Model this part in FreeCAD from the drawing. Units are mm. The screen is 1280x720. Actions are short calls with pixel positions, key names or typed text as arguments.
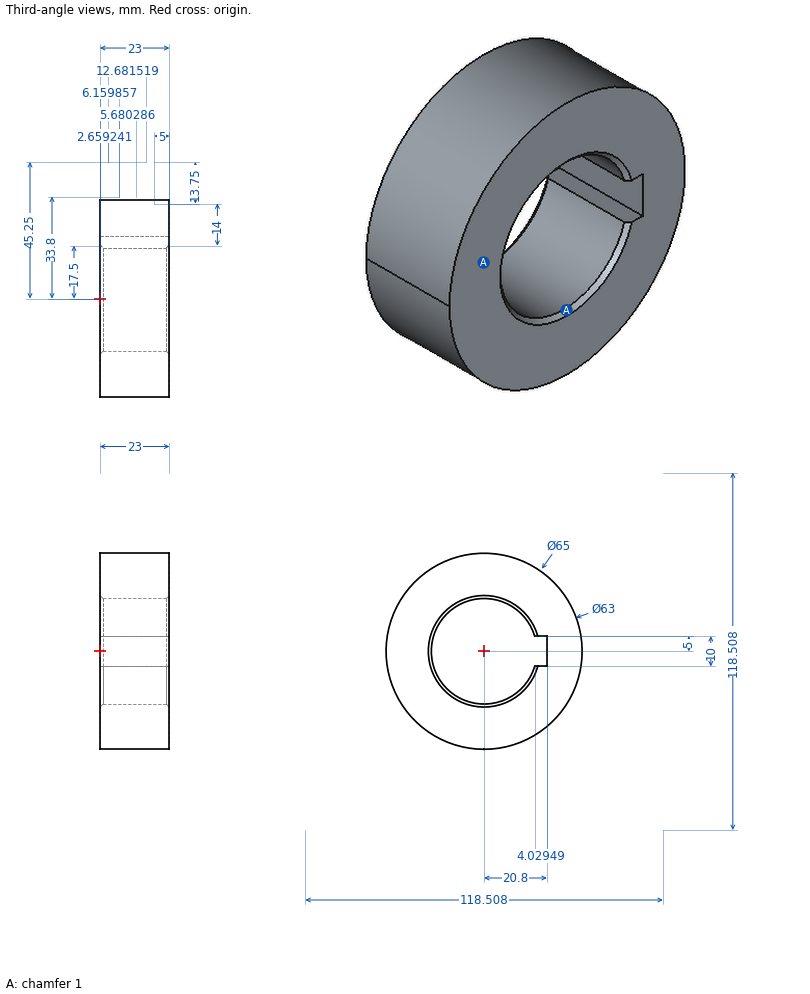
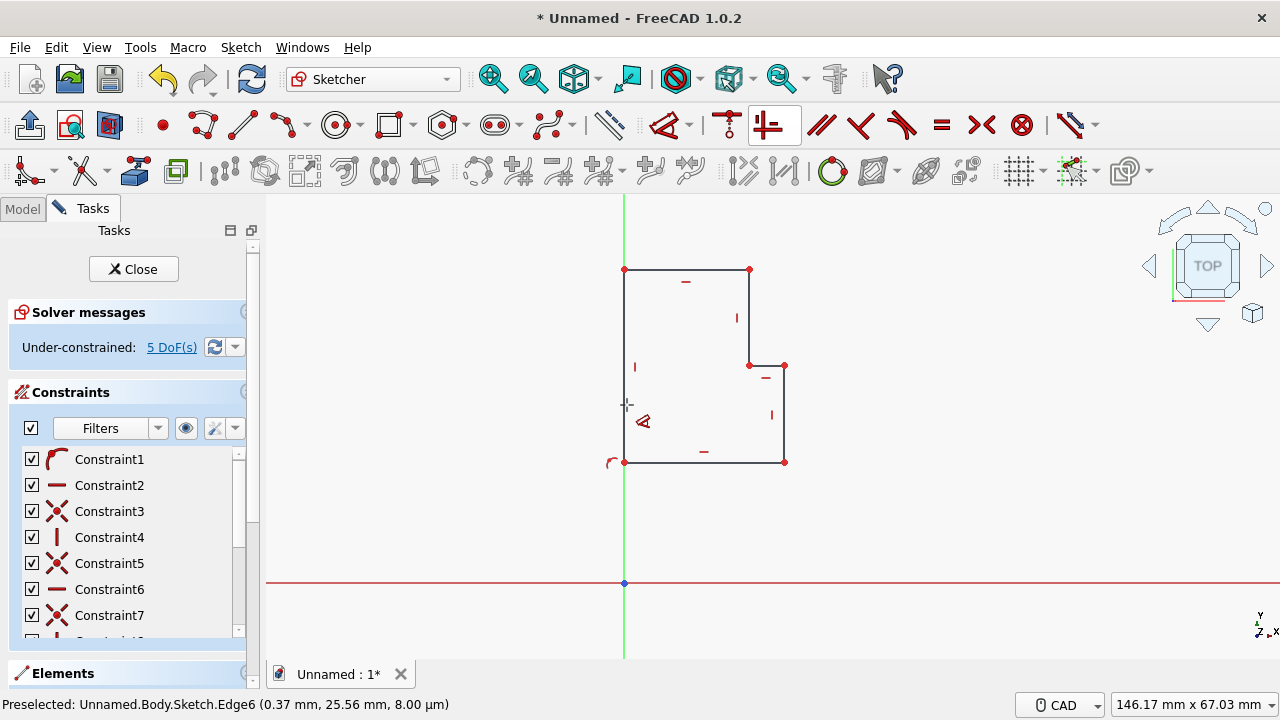
scroll(773, 366, up, 2)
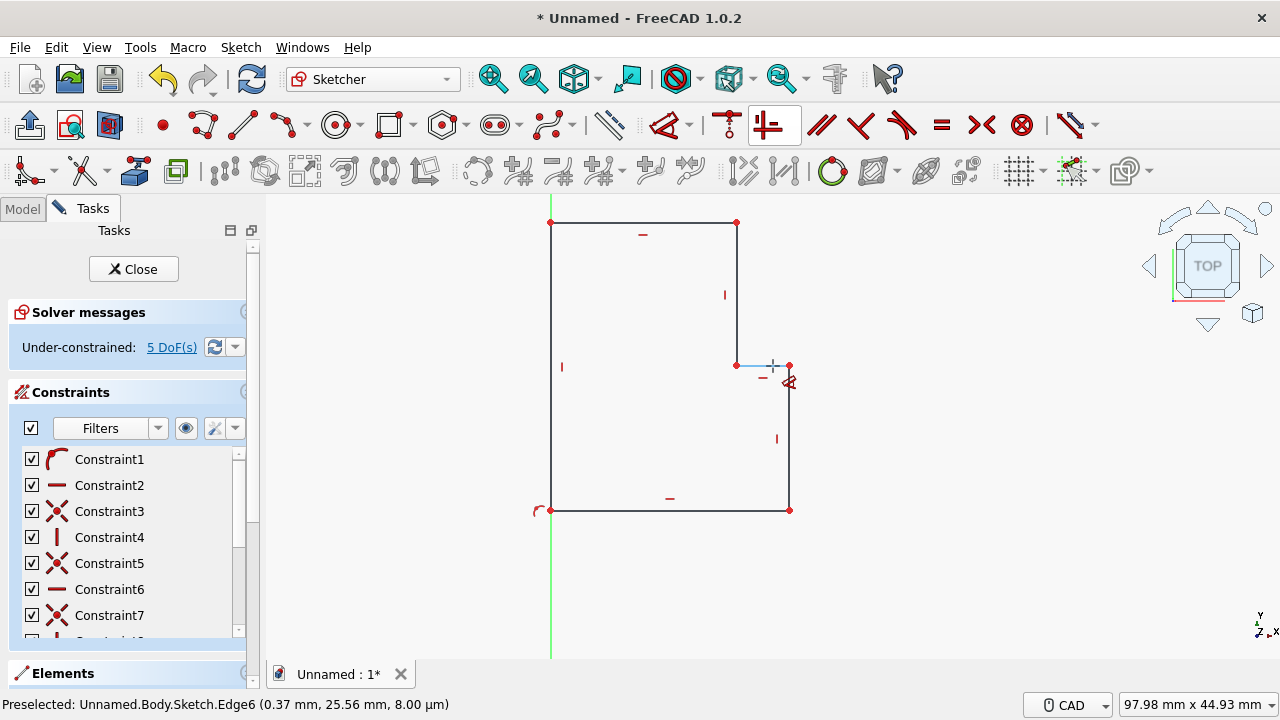
click(773, 366)
click(763, 332)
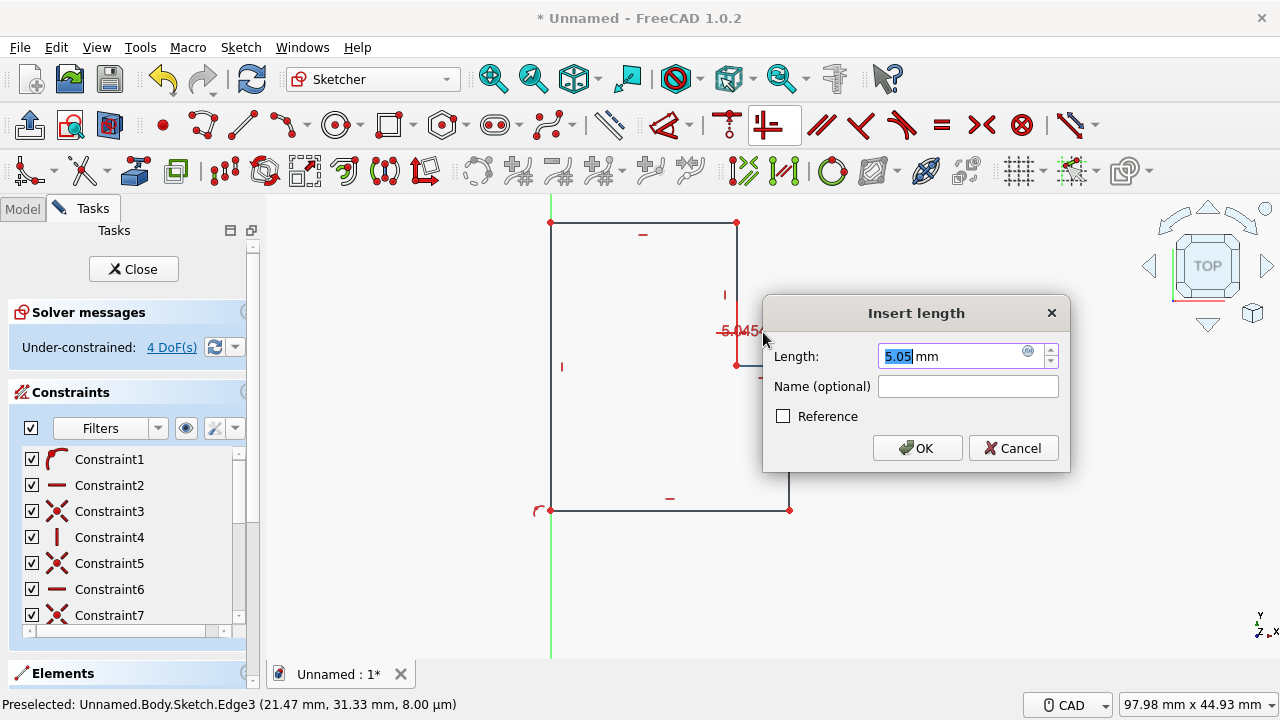
text(5)
key(Return)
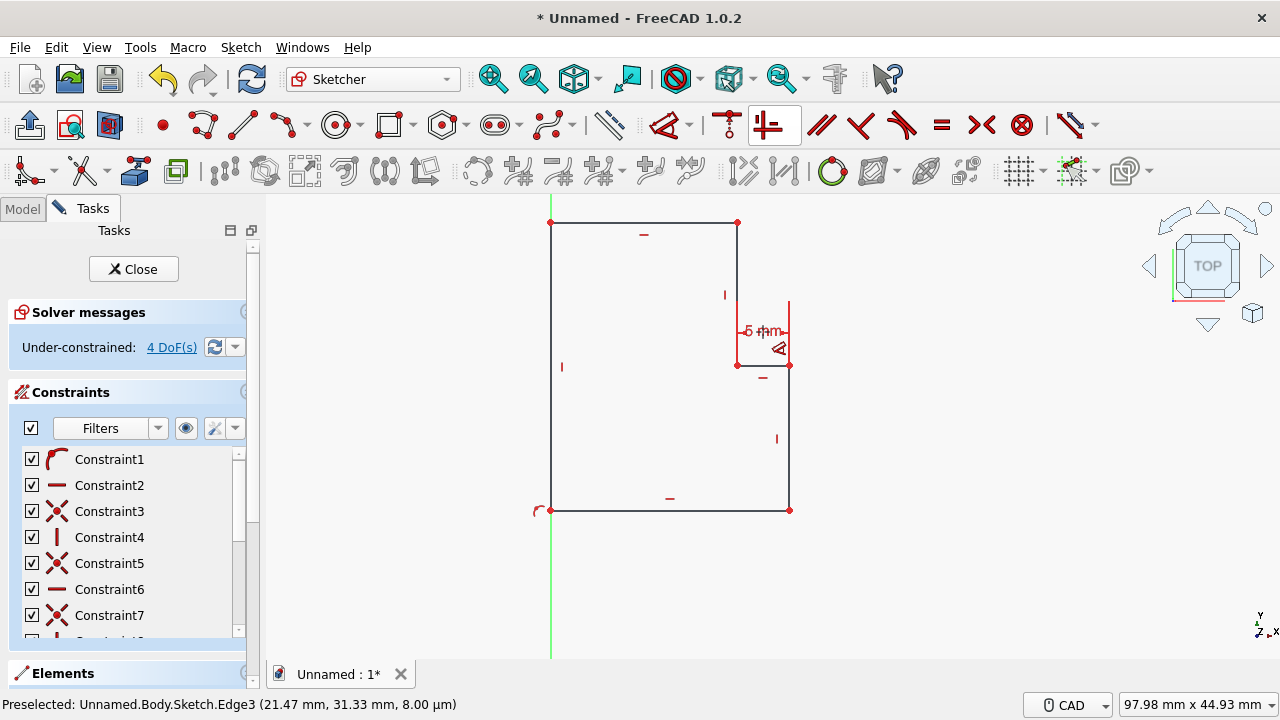
click(622, 511)
click(670, 545)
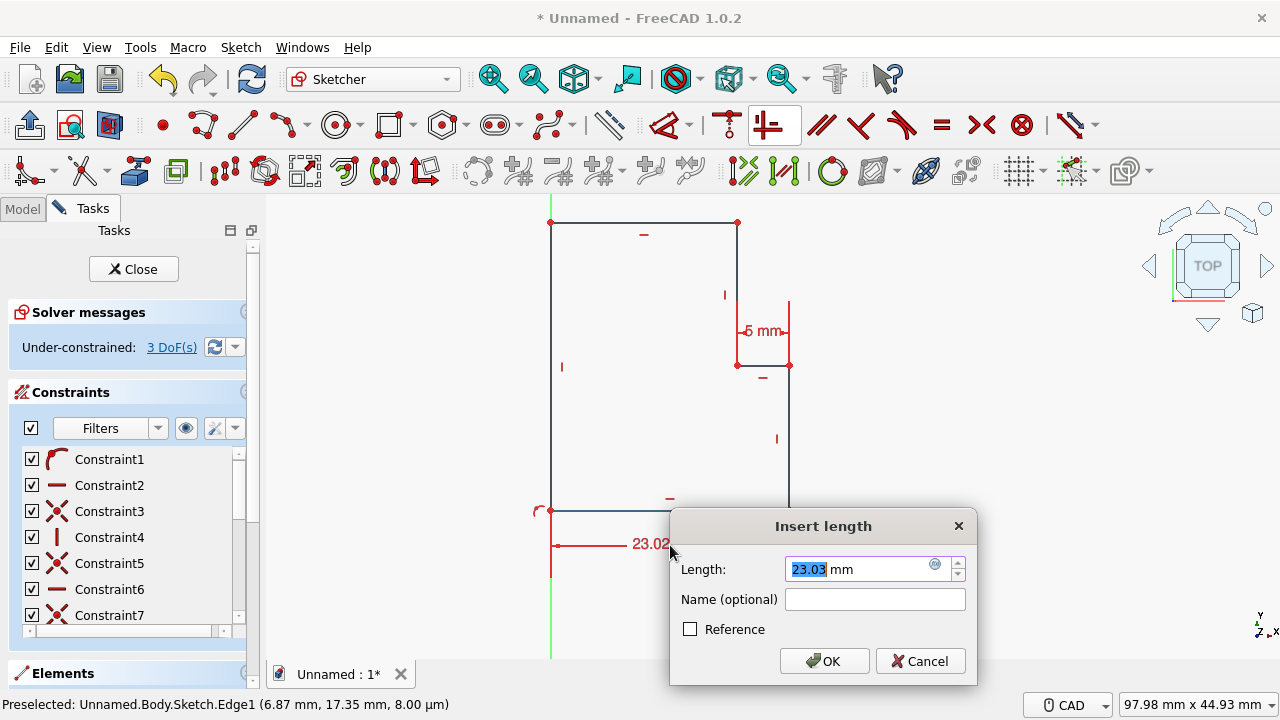
text(23)
key(Return)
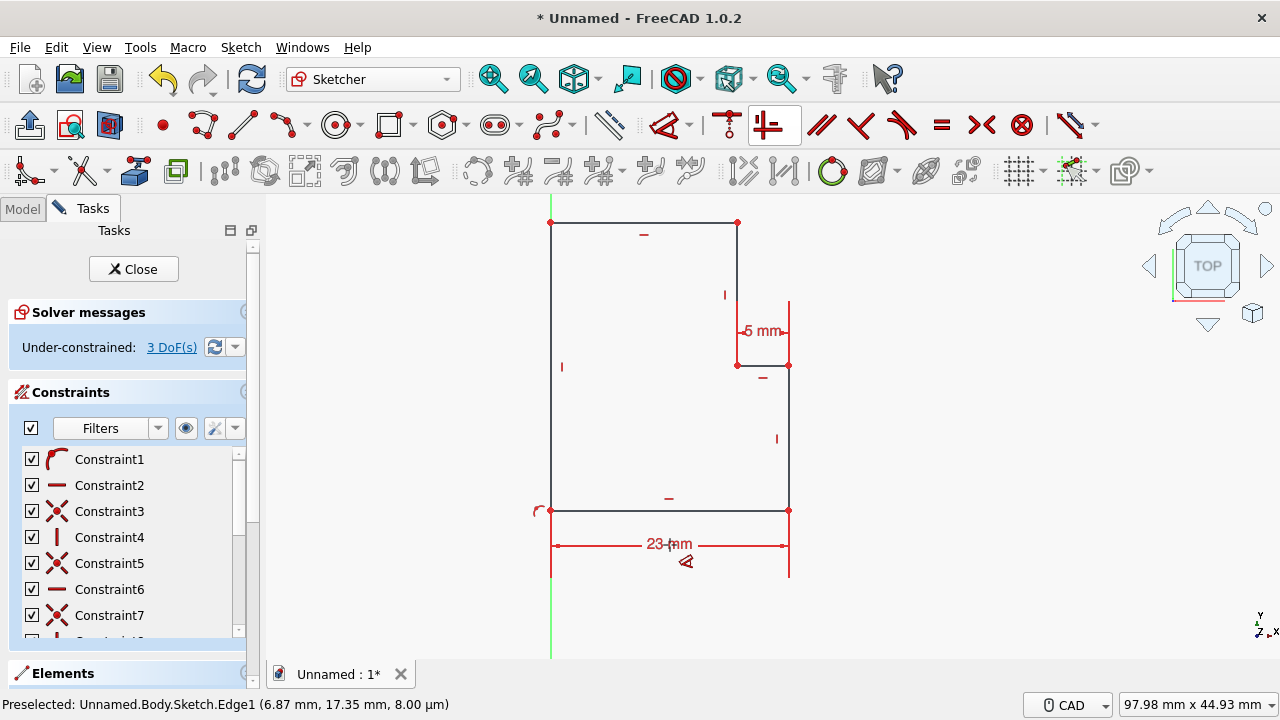
click(789, 467)
click(823, 438)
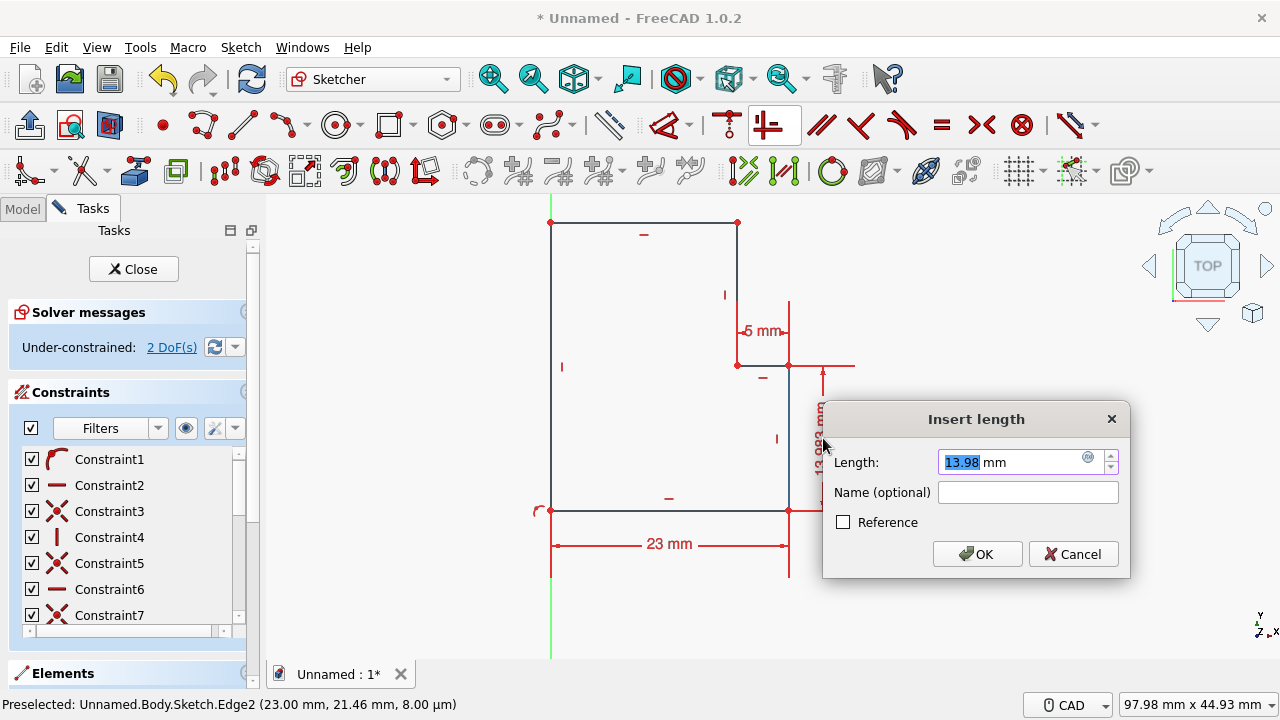
text(14)
key(Return)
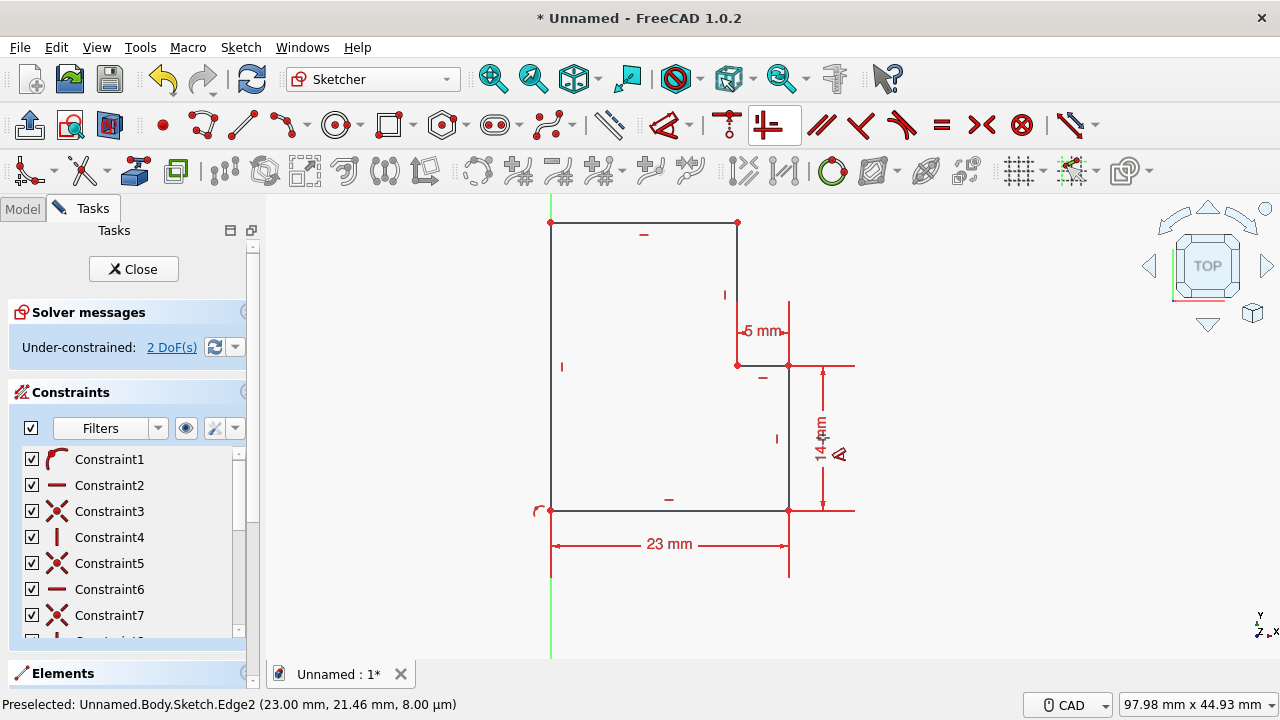
click(737, 323)
click(771, 294)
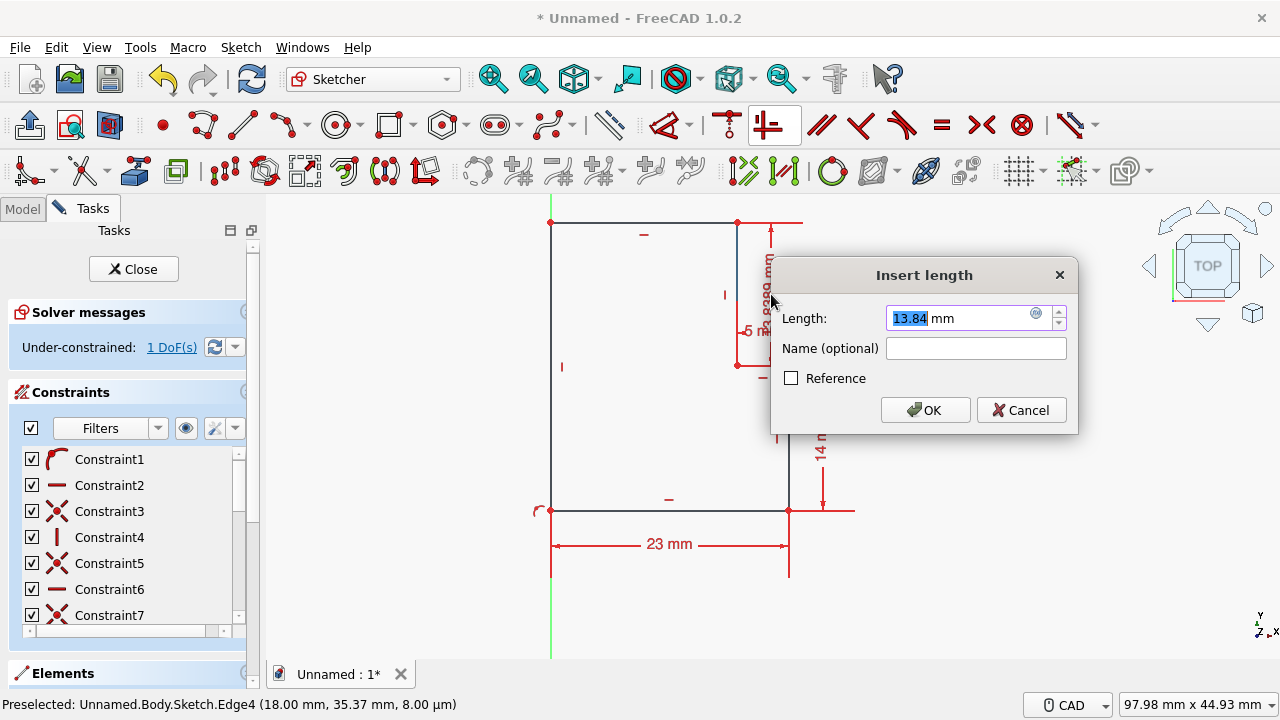
text(13.75)
key(Return)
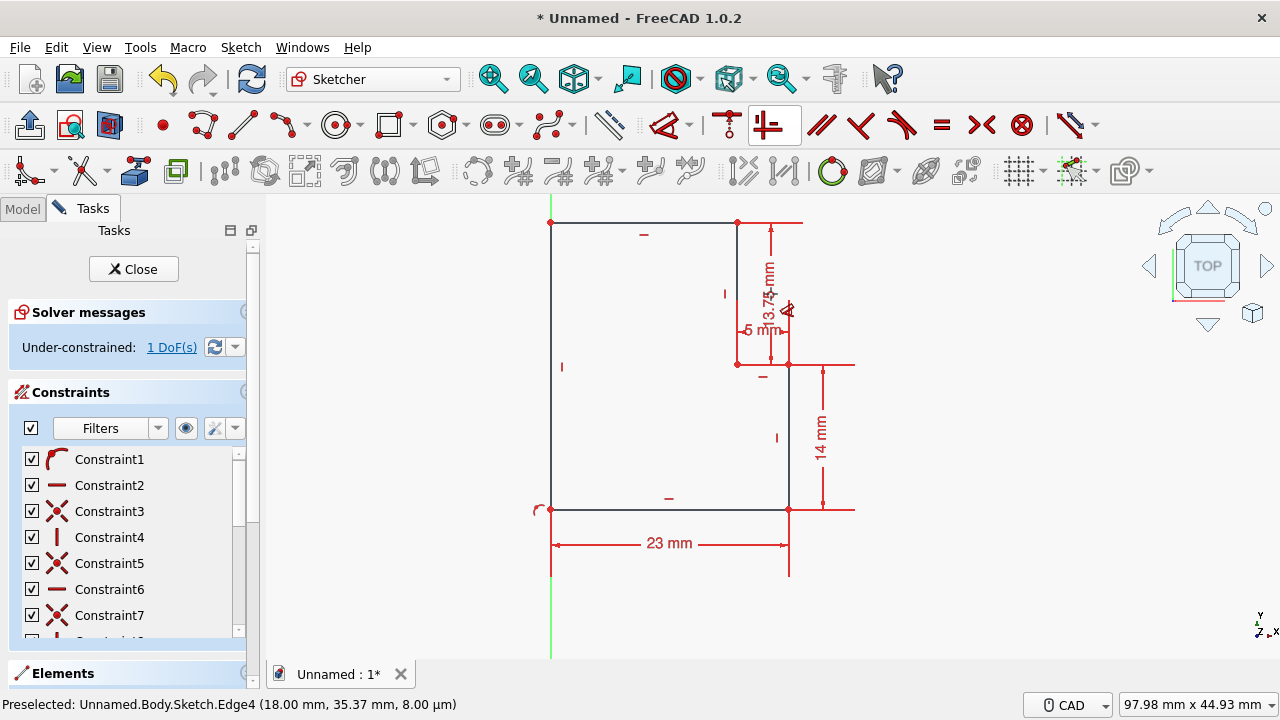
click(551, 510)
click(517, 570)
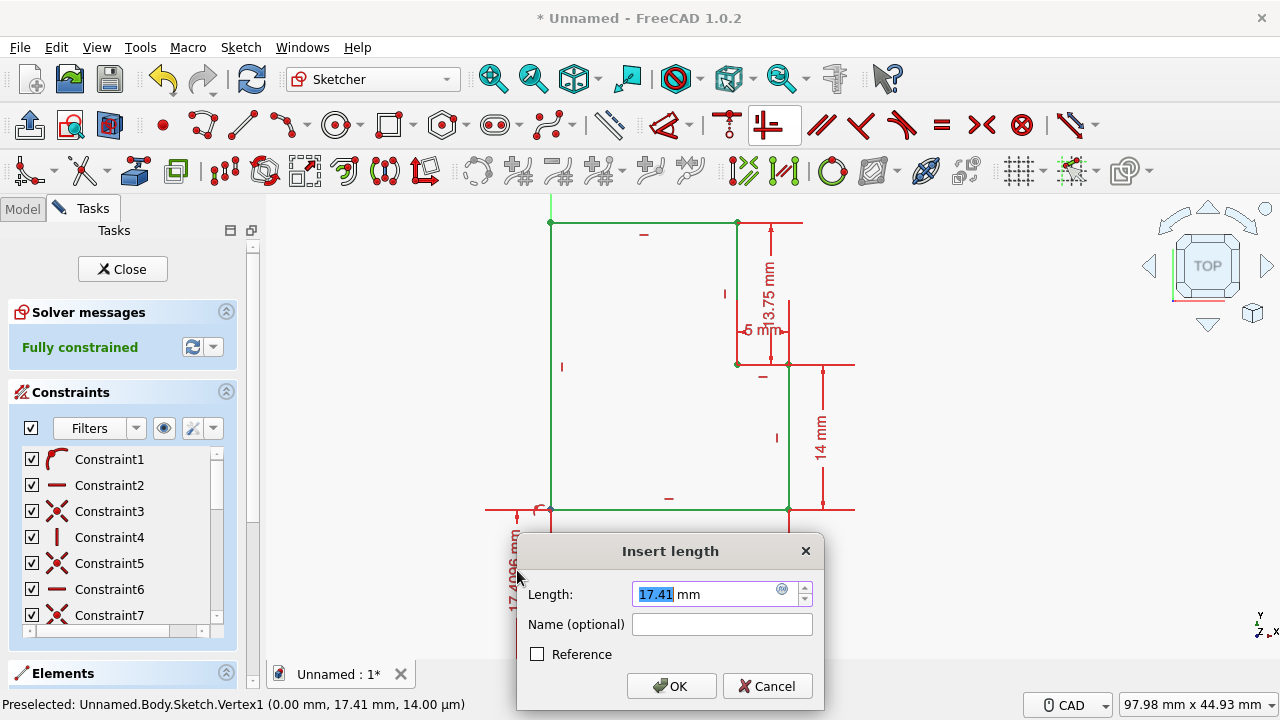
text(17.5)
key(Return)
key(Escape)